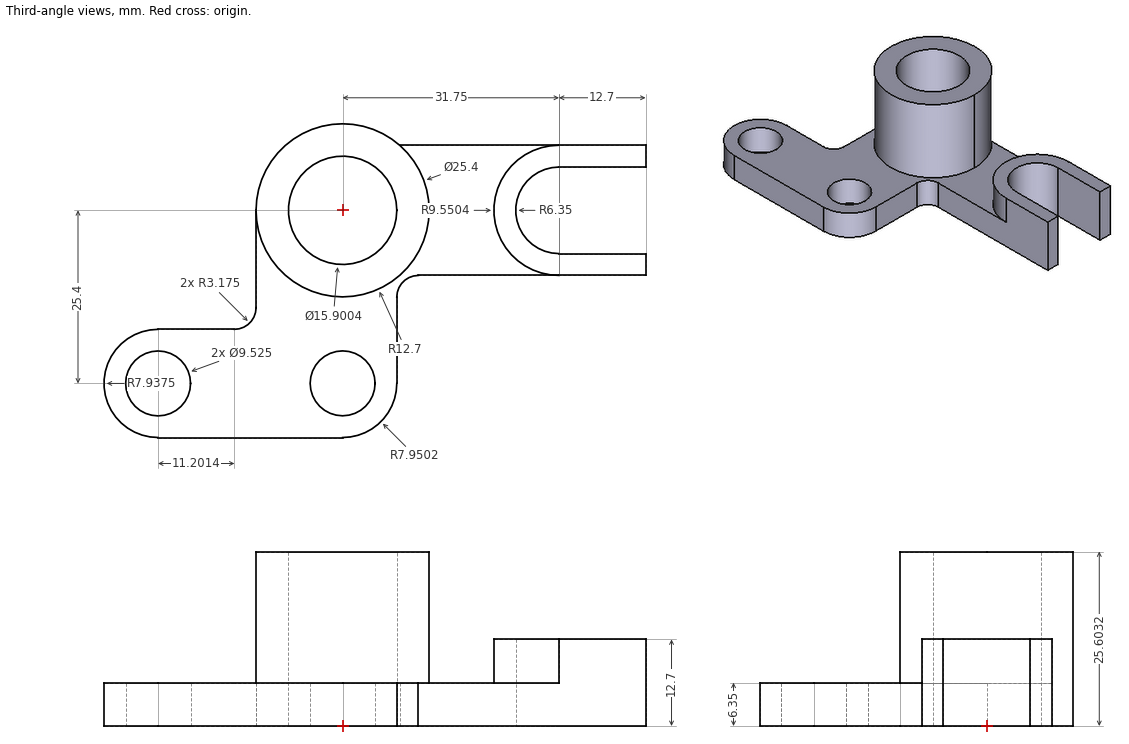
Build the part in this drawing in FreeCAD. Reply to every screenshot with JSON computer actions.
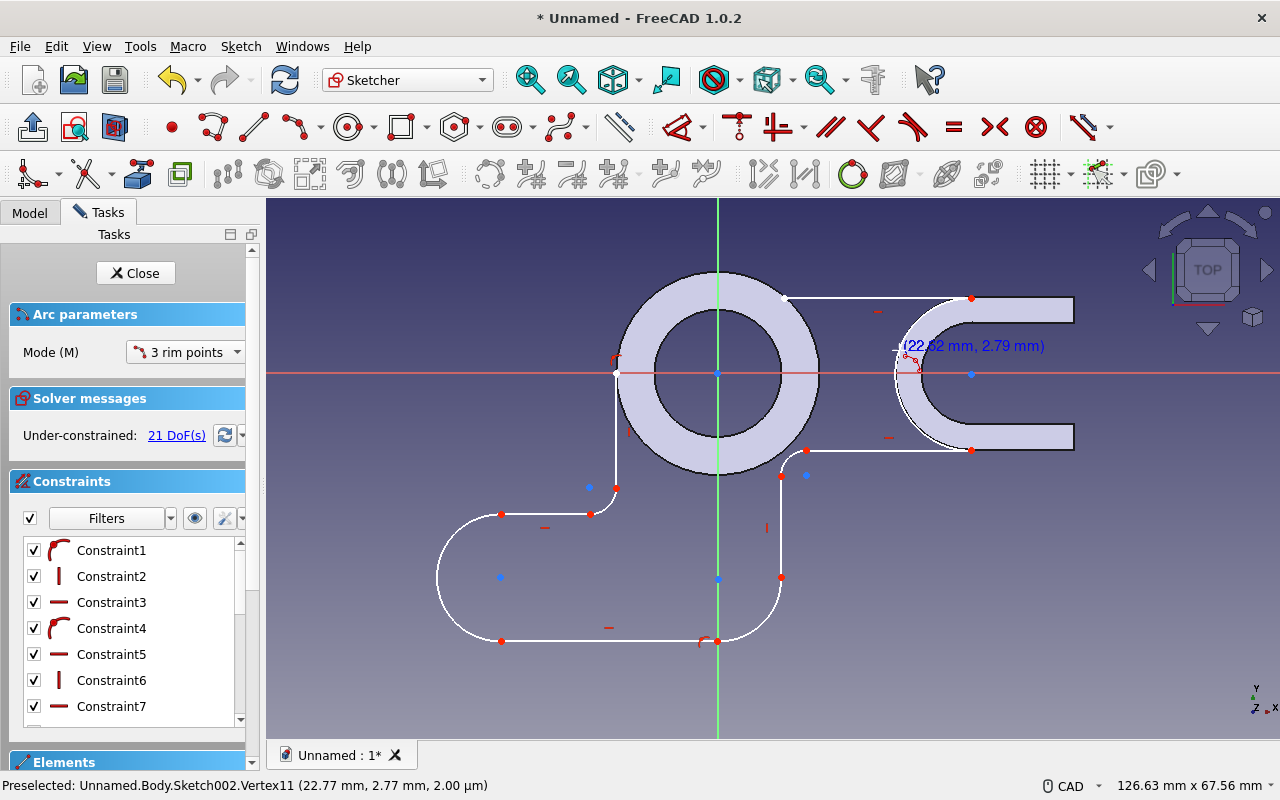
{"action": "left_click", "coordinate": [785, 298]}
{"action": "left_click", "coordinate": [616, 373]}
{"action": "left_click", "coordinate": [760, 466]}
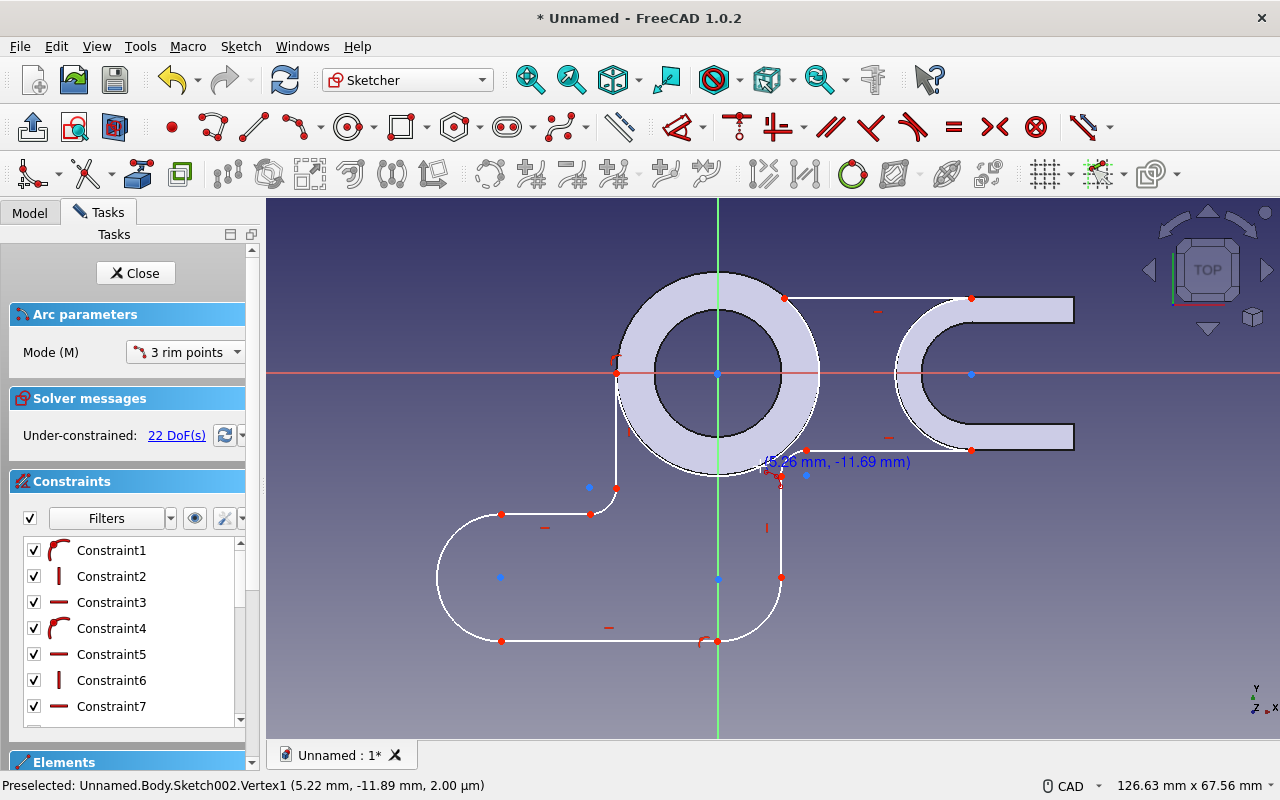
{"action": "left_click", "coordinate": [348, 128]}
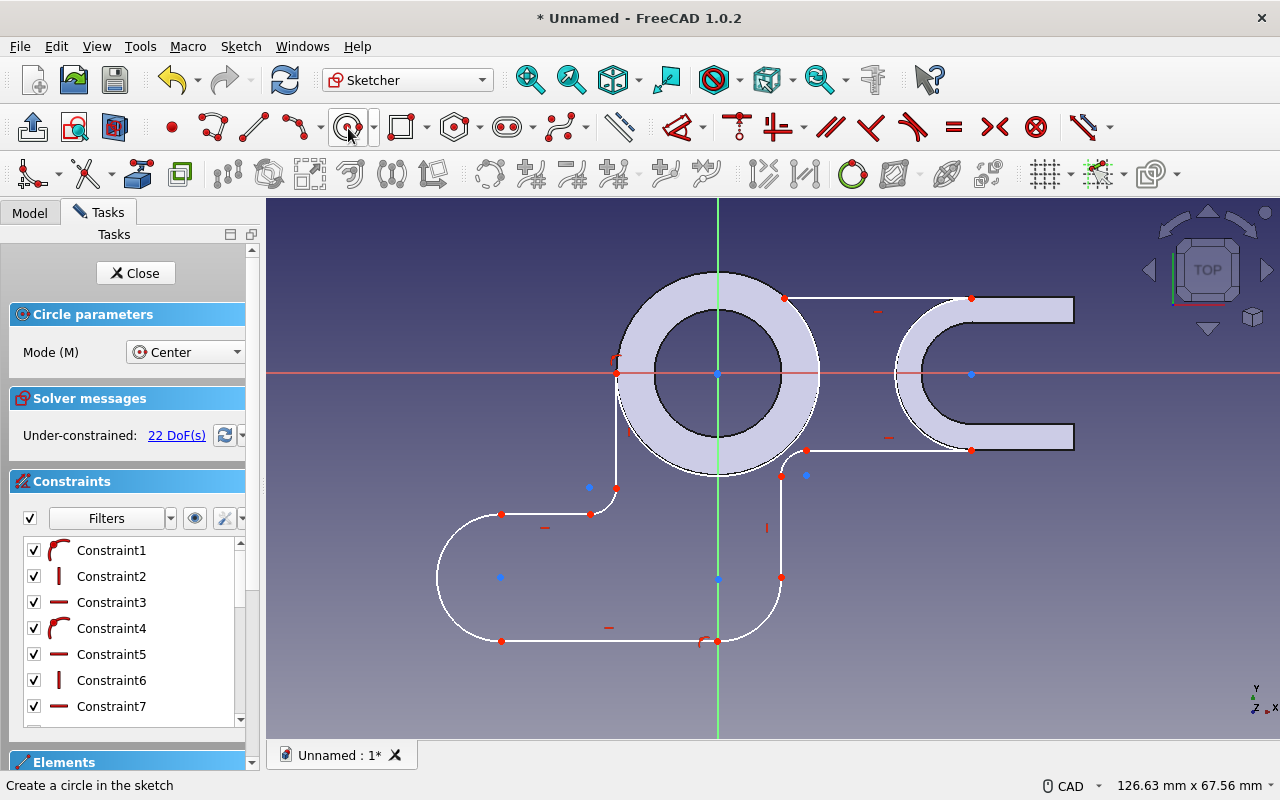
{"action": "left_click", "coordinate": [501, 577]}
{"action": "left_click", "coordinate": [528, 550]}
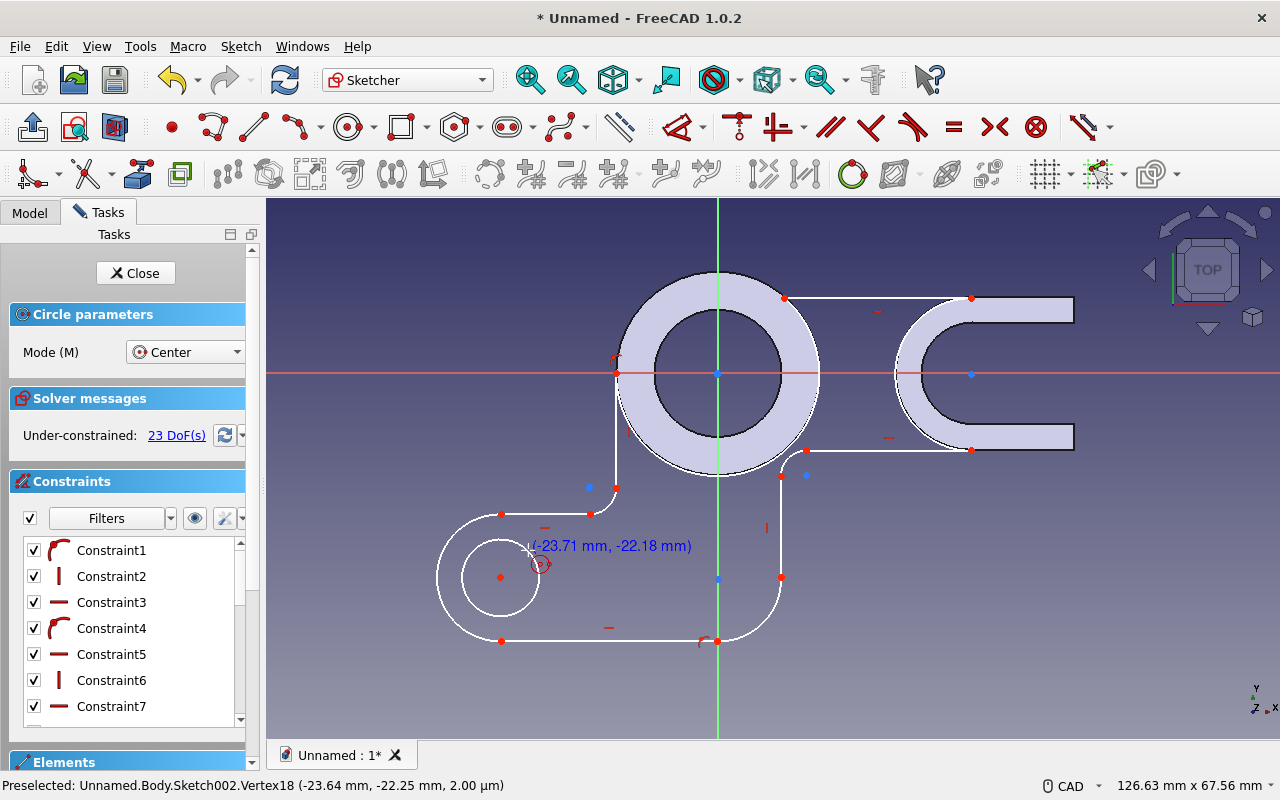
{"action": "left_click", "coordinate": [718, 577]}
{"action": "left_click", "coordinate": [745, 550]}
{"action": "key", "text": "Escape"}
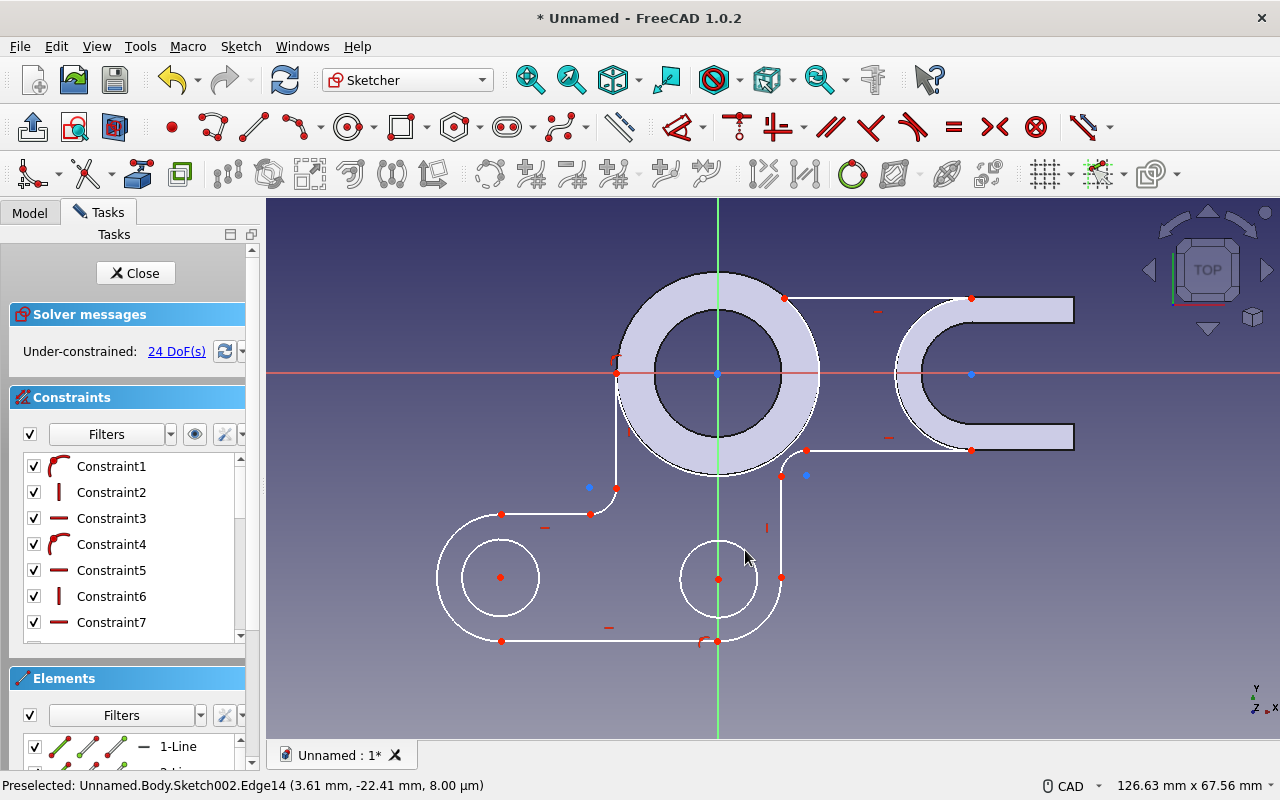
{"action": "left_click", "coordinate": [616, 454]}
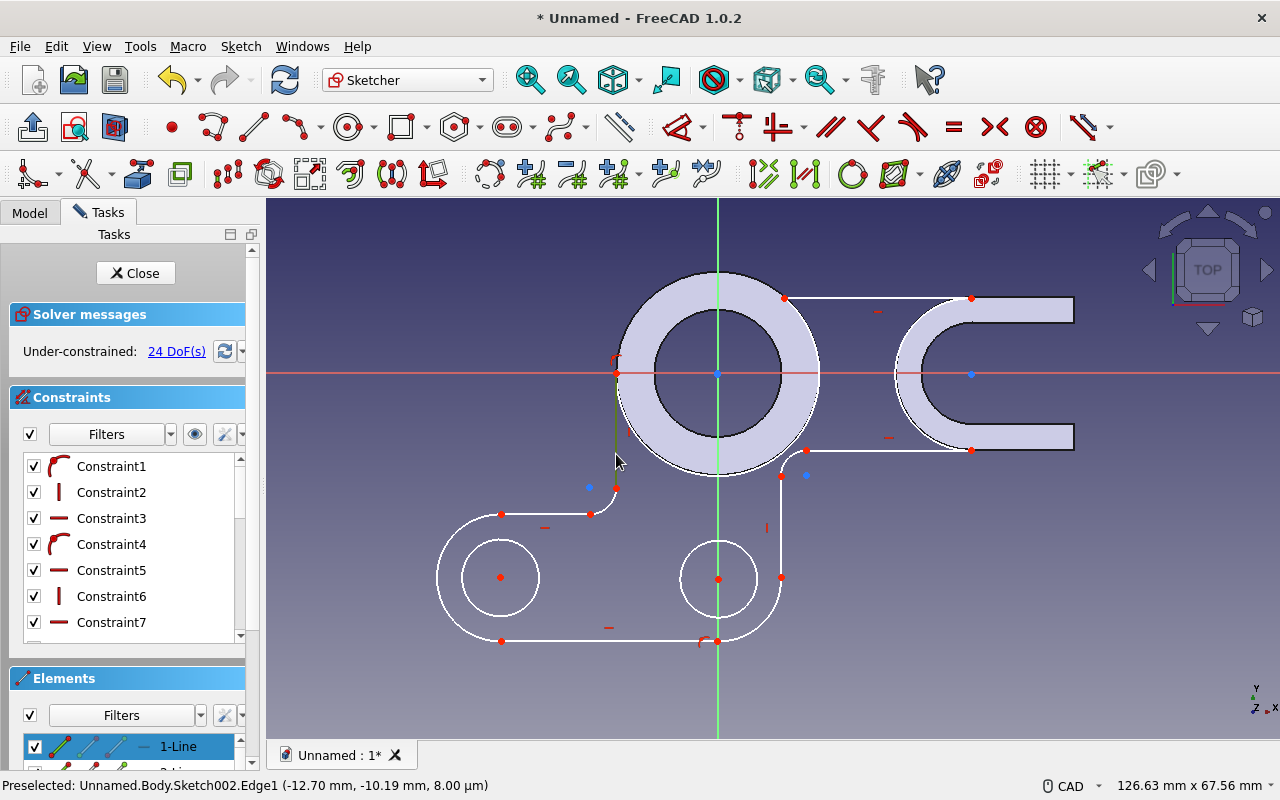
{"action": "left_click", "coordinate": [602, 511]}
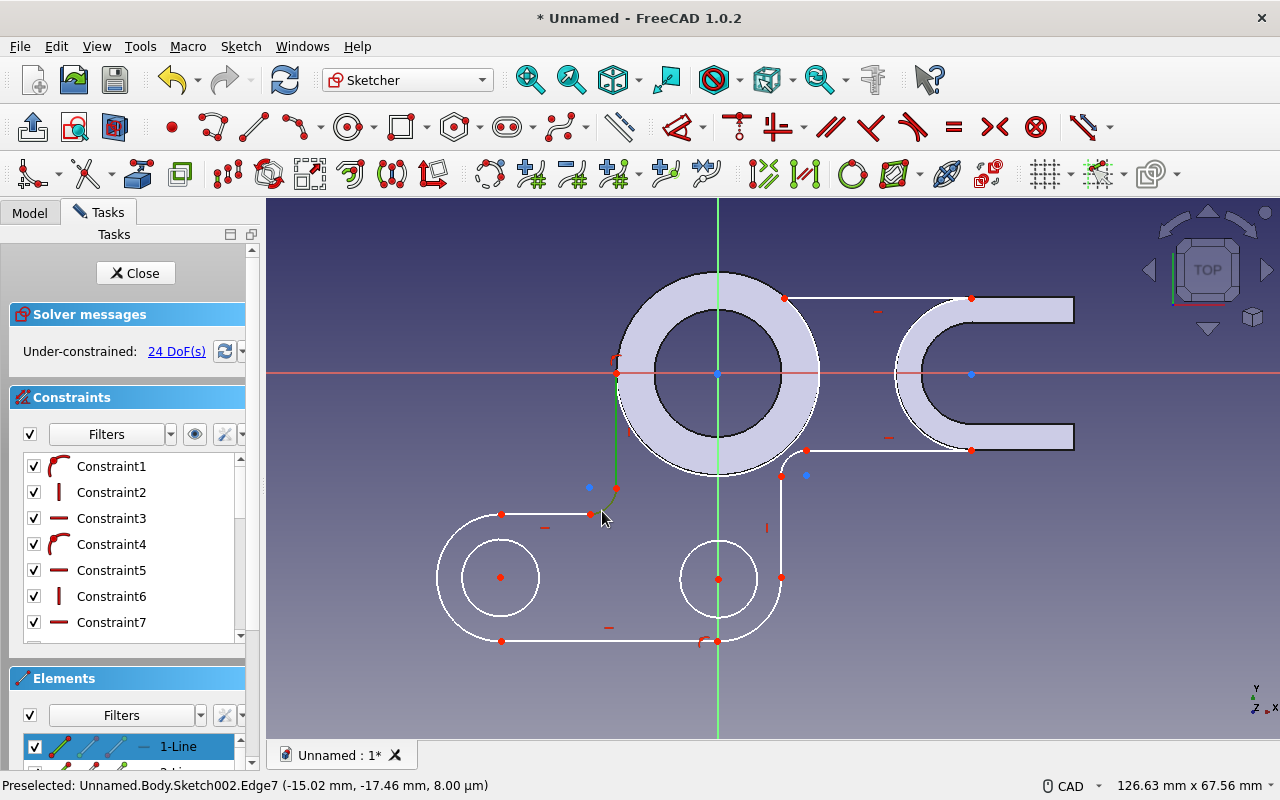
{"action": "left_click", "coordinate": [913, 128]}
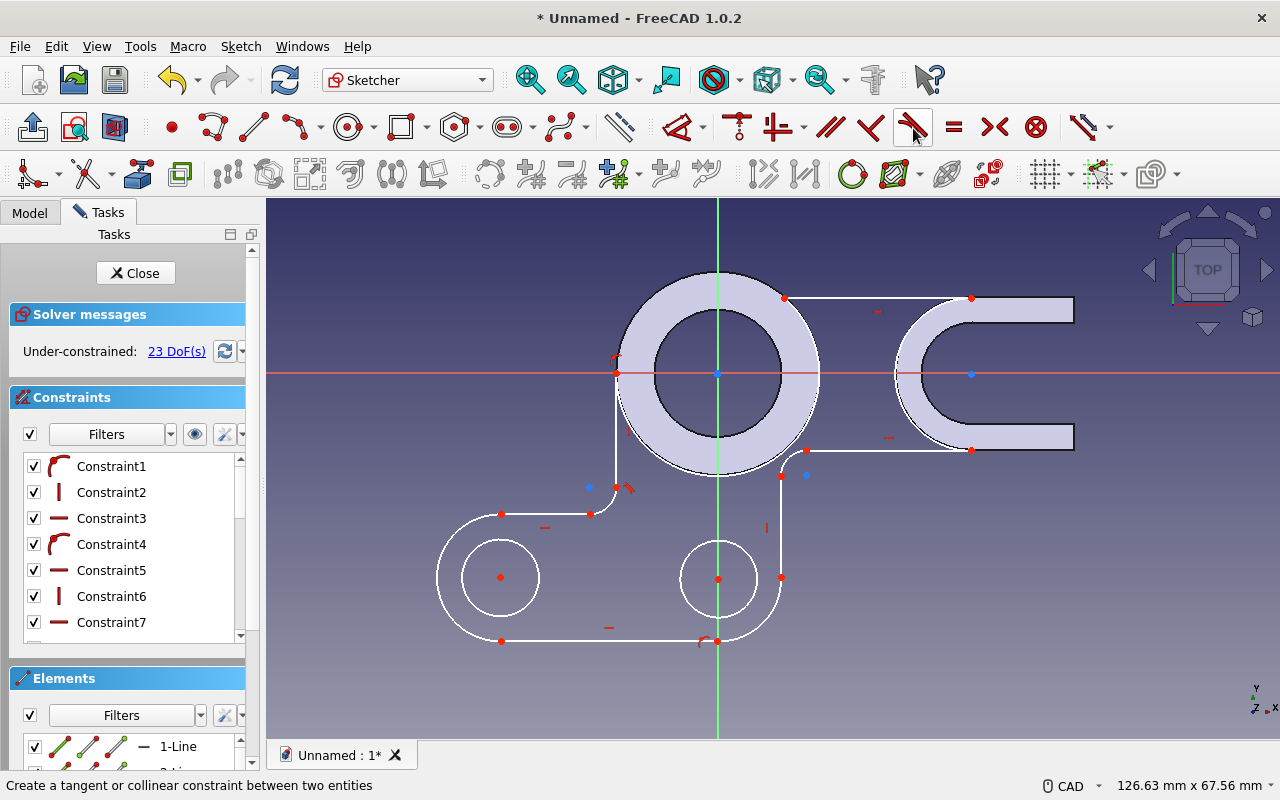
{"action": "left_click", "coordinate": [616, 453]}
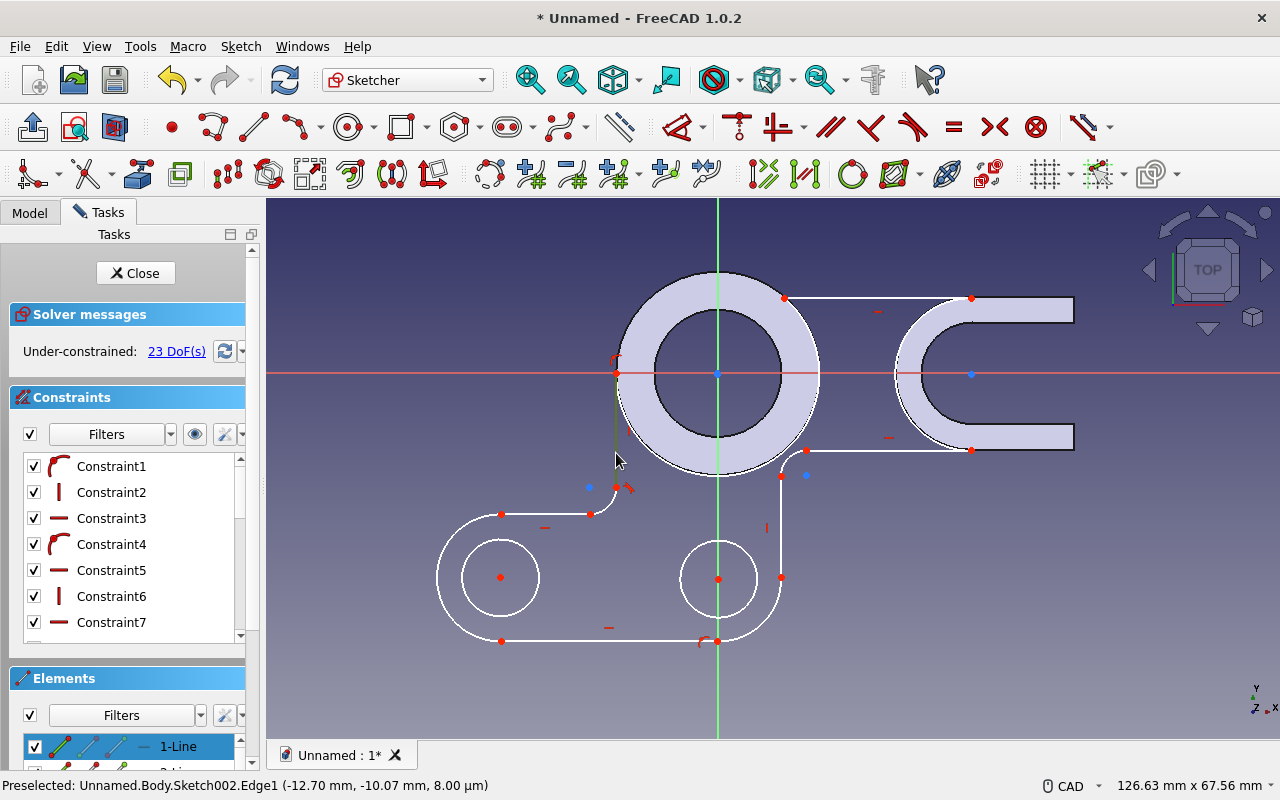
{"action": "left_click", "coordinate": [680, 469]}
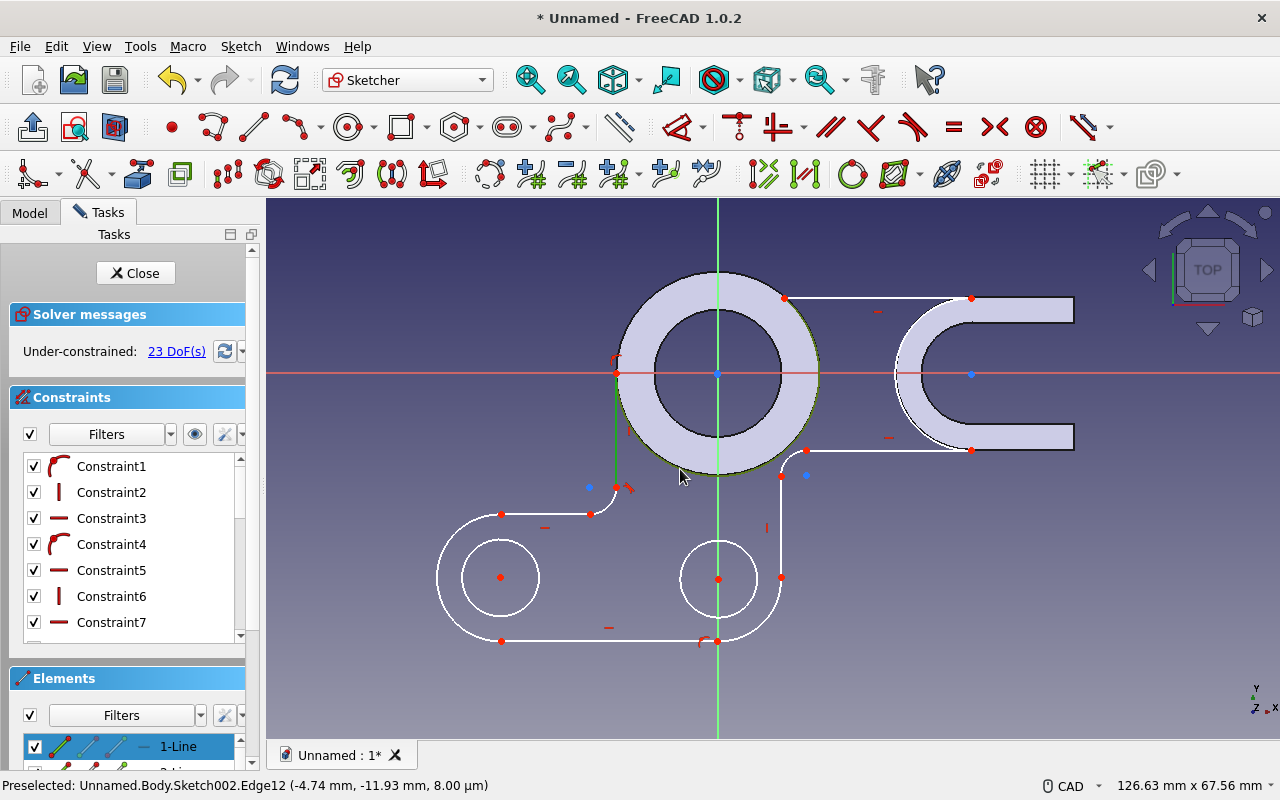
{"action": "left_click", "coordinate": [913, 128]}